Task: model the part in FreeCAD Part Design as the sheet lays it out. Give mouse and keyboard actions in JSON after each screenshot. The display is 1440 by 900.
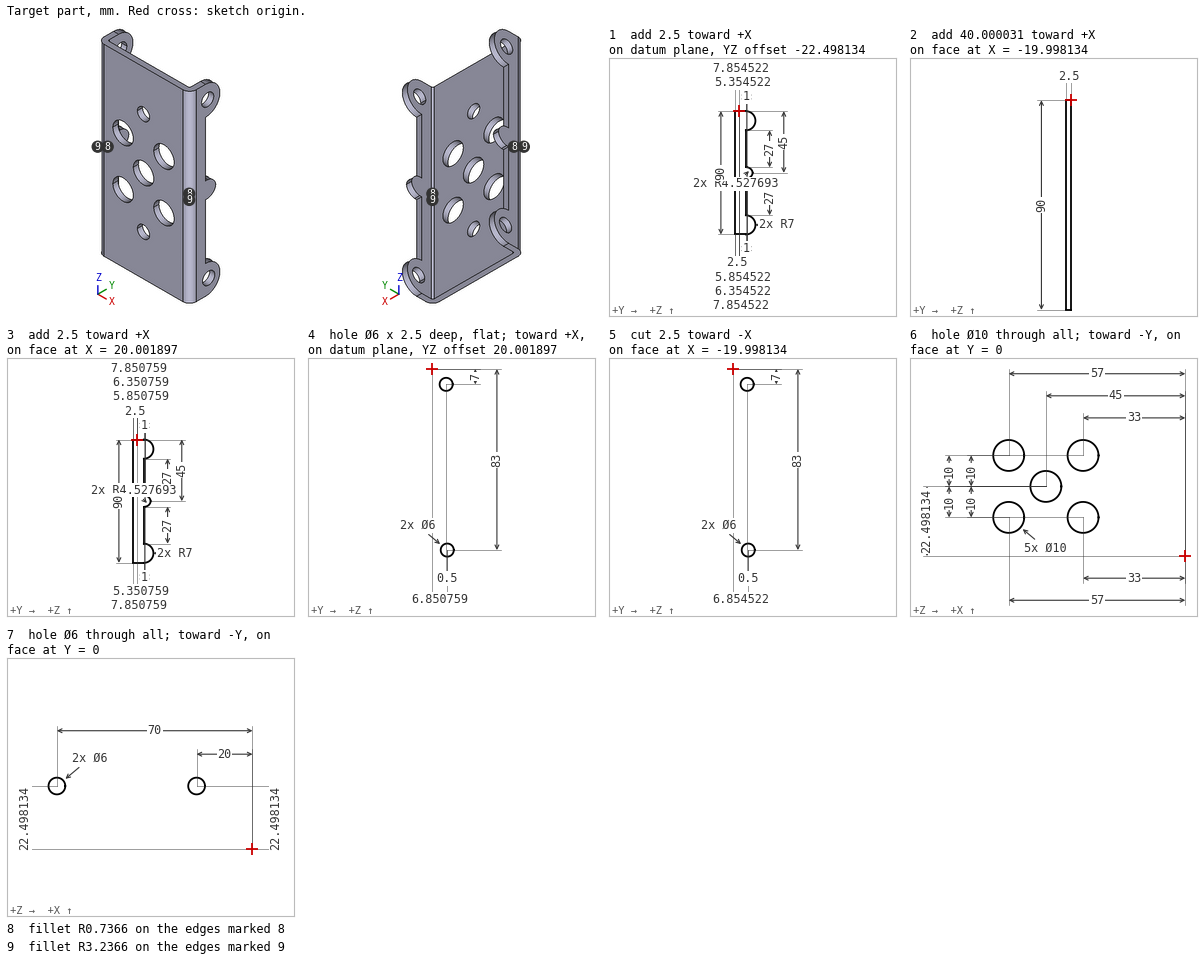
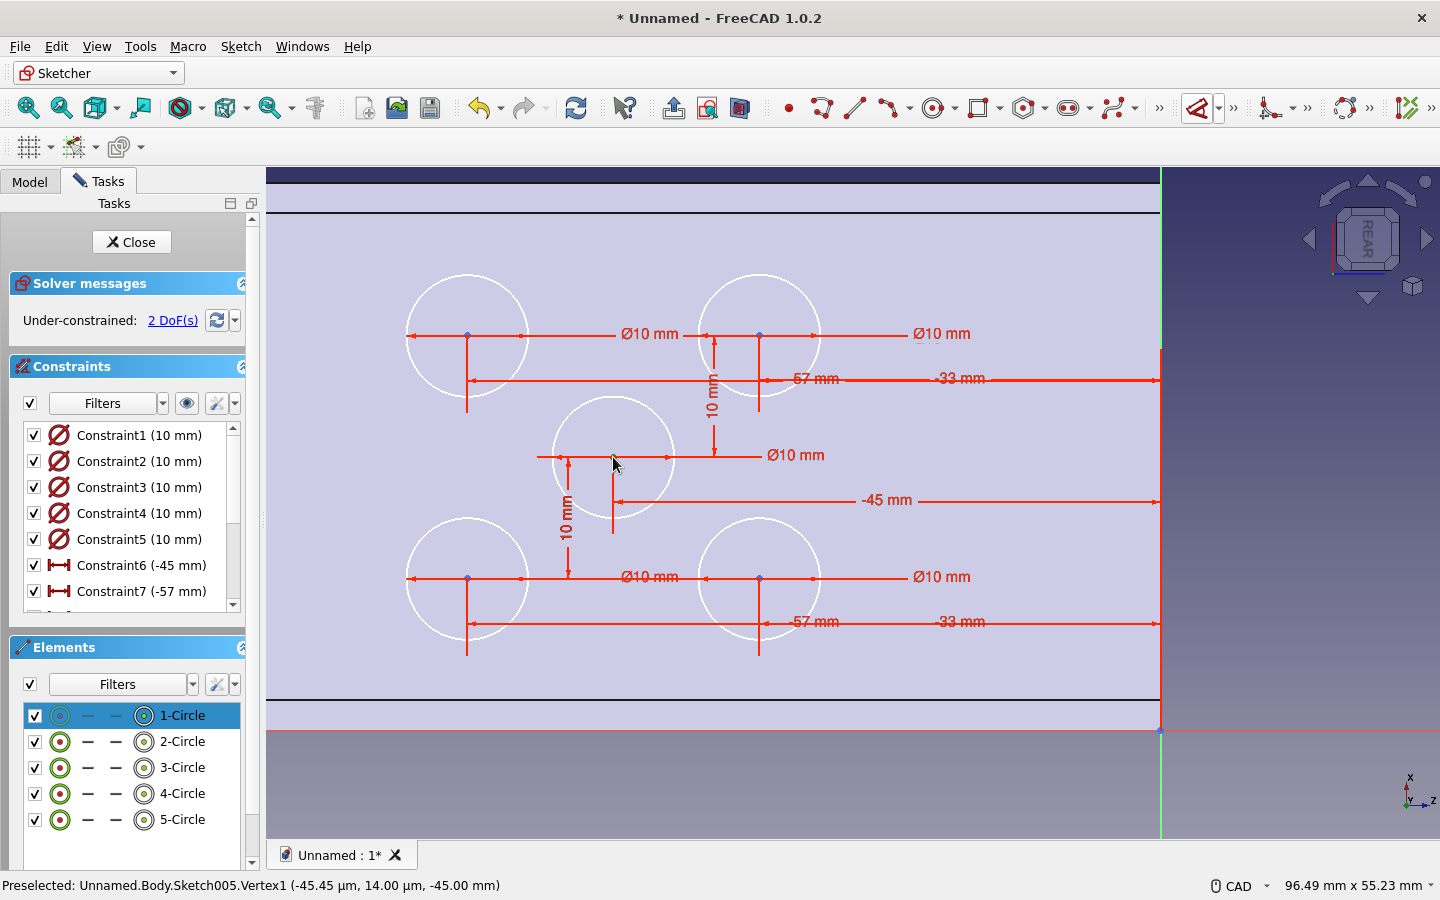
{"action": "left_click", "coordinate": [467, 336]}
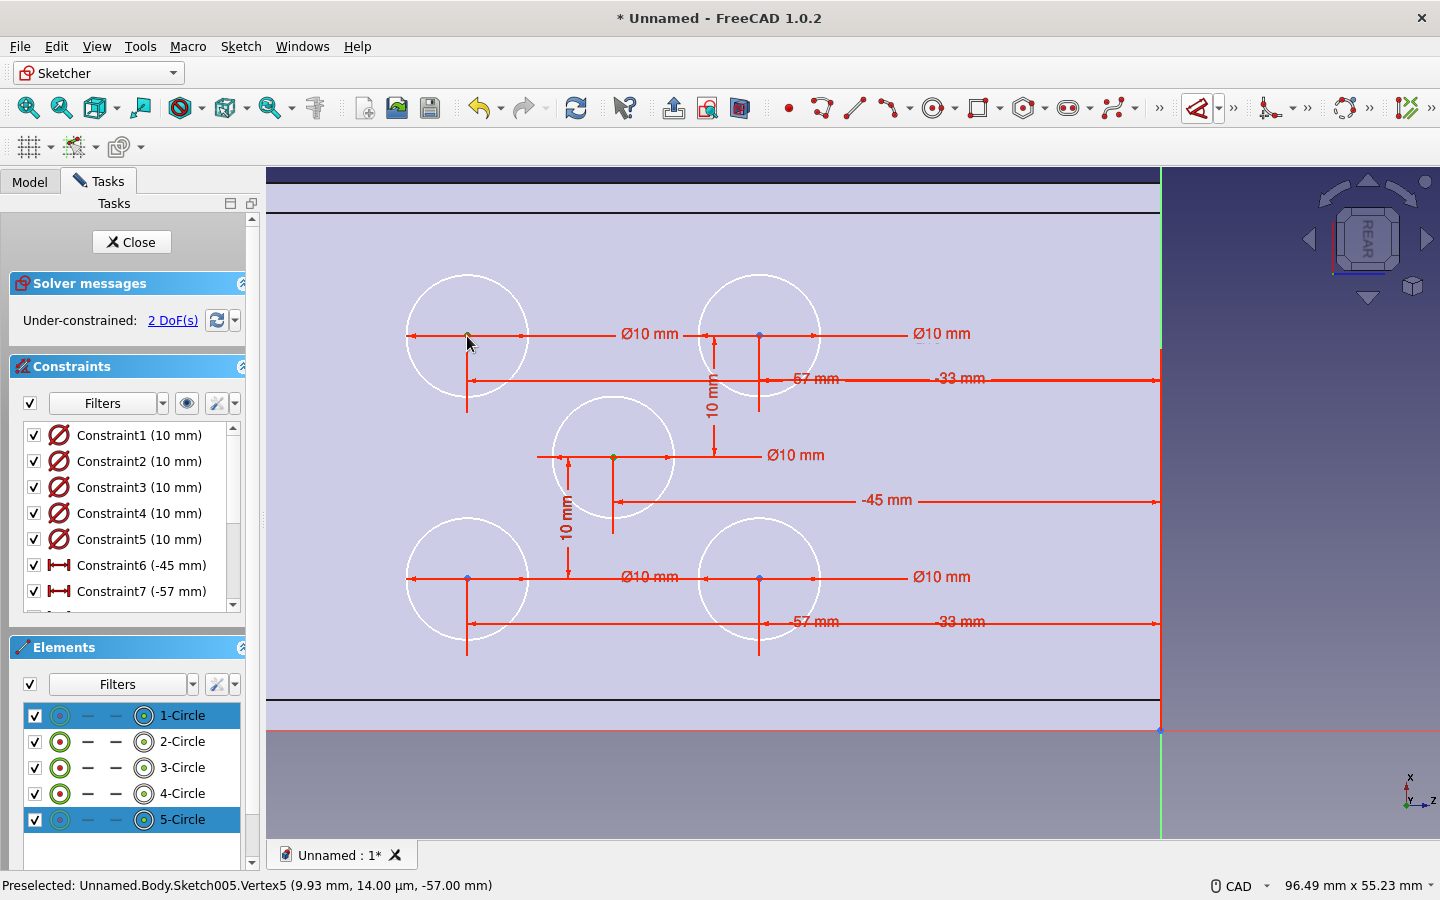
{"action": "key", "text": "i"}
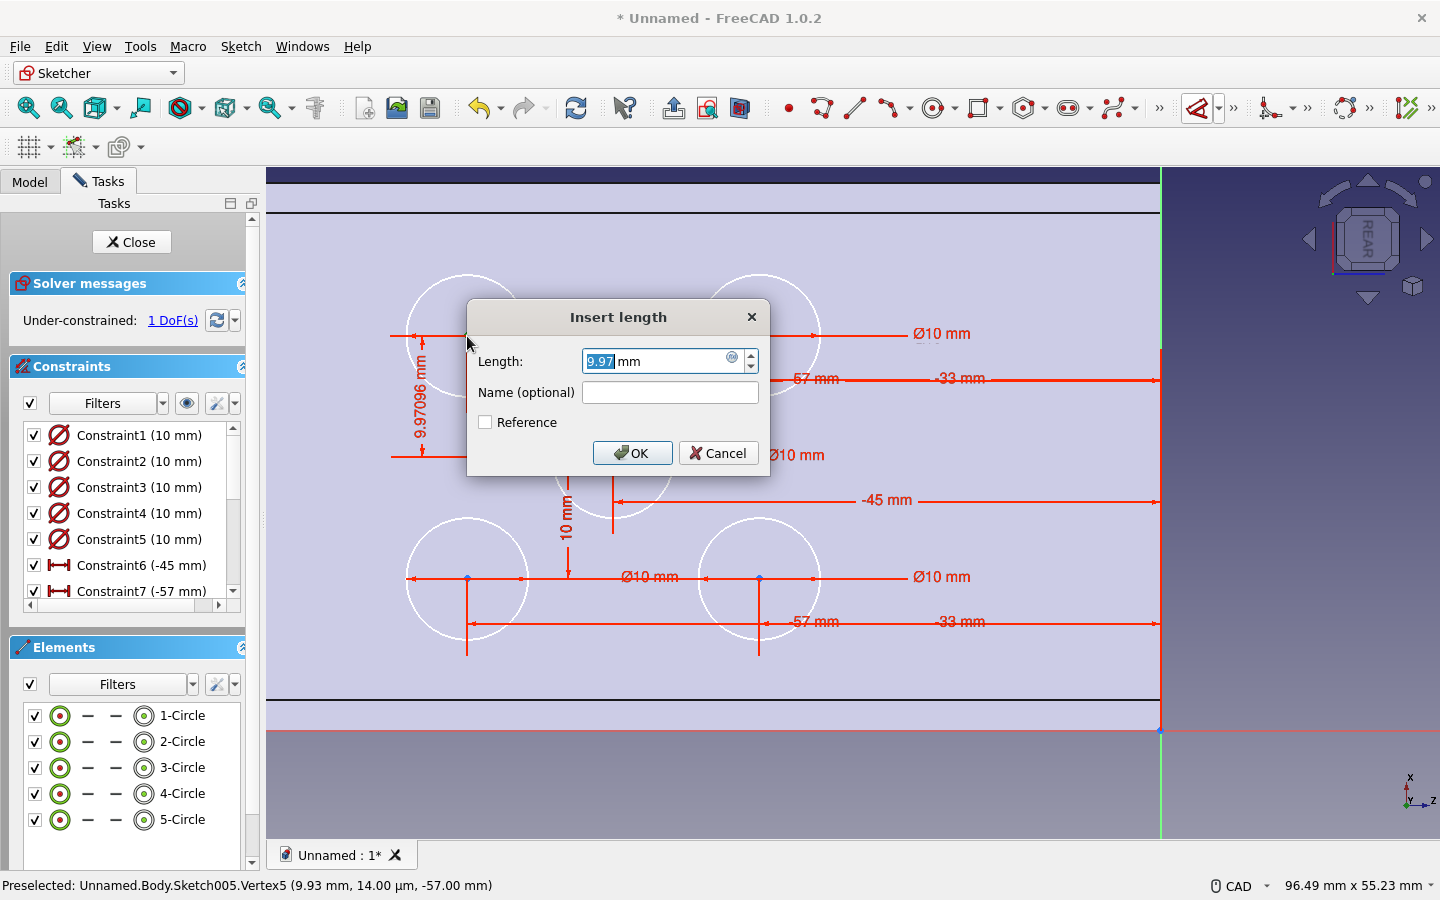
{"action": "type", "text": "10"}
{"action": "key", "text": "Return"}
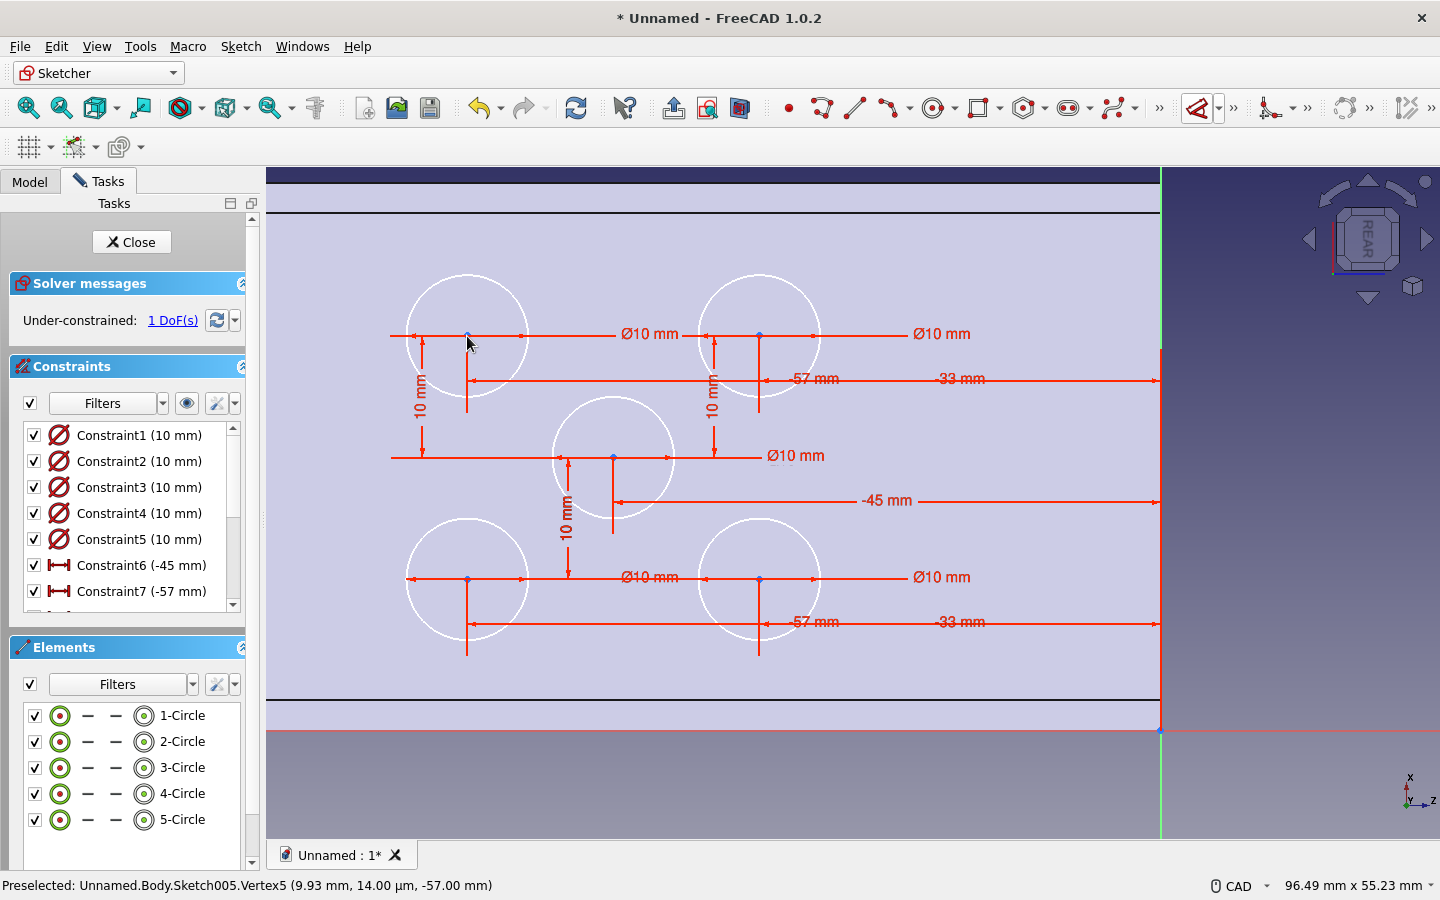
{"action": "left_click", "coordinate": [613, 458]}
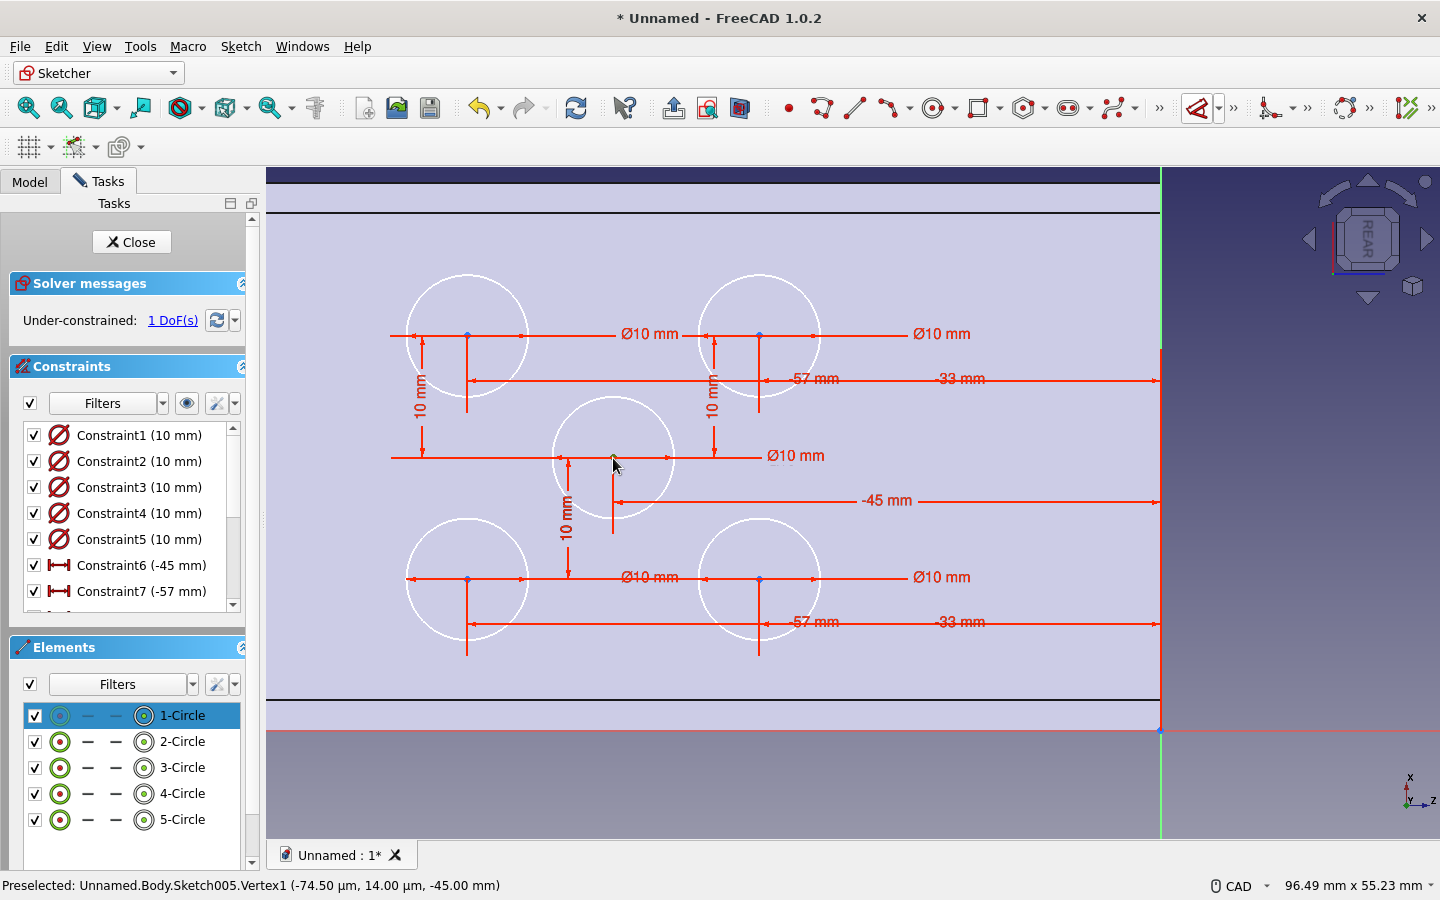
{"action": "left_click", "coordinate": [1218, 108]}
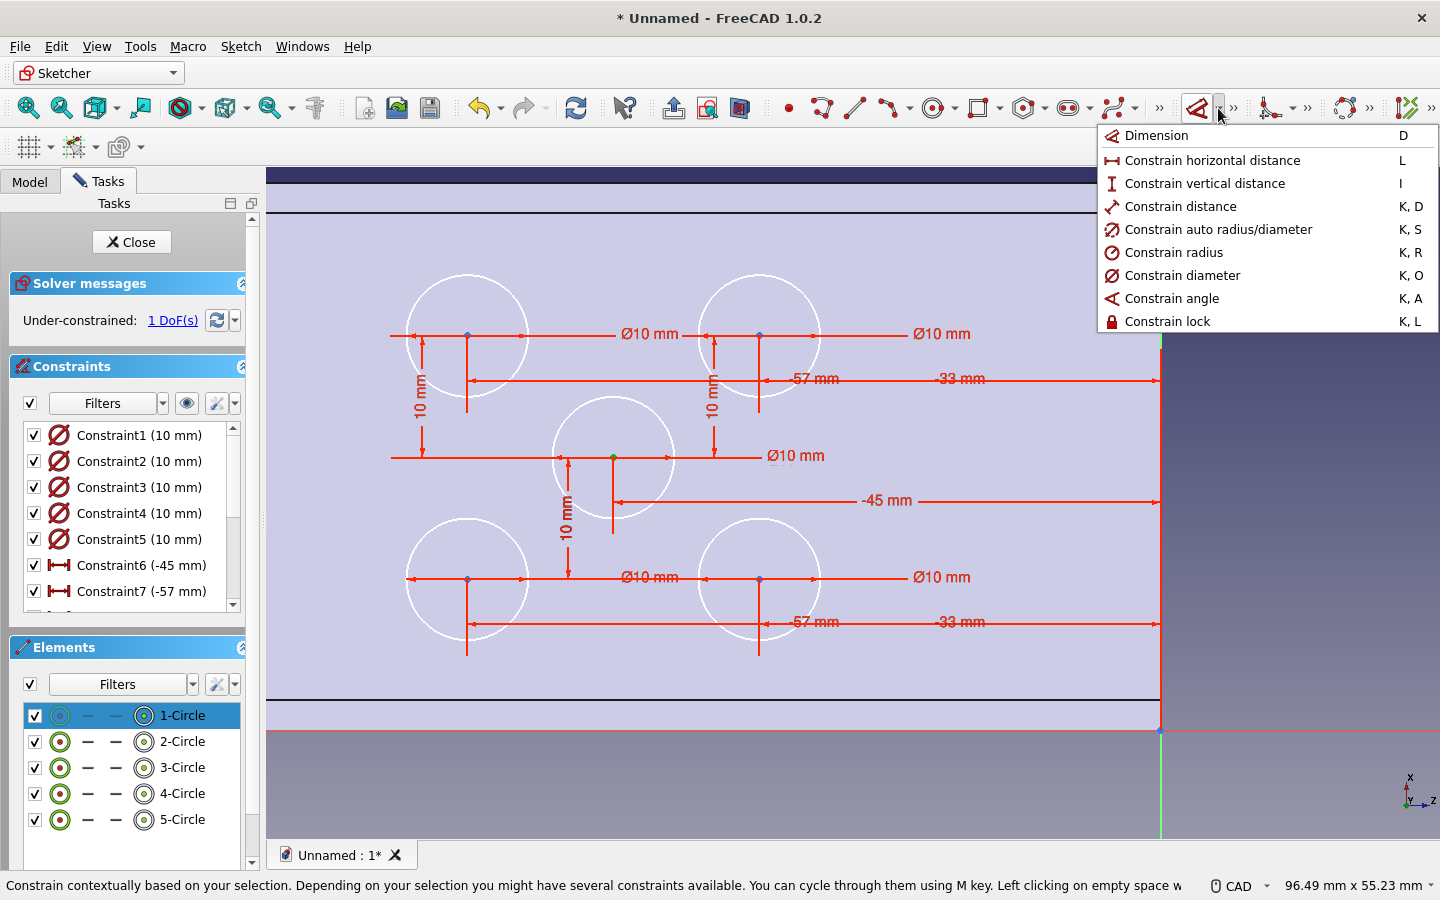
{"action": "left_click", "coordinate": [1268, 184]}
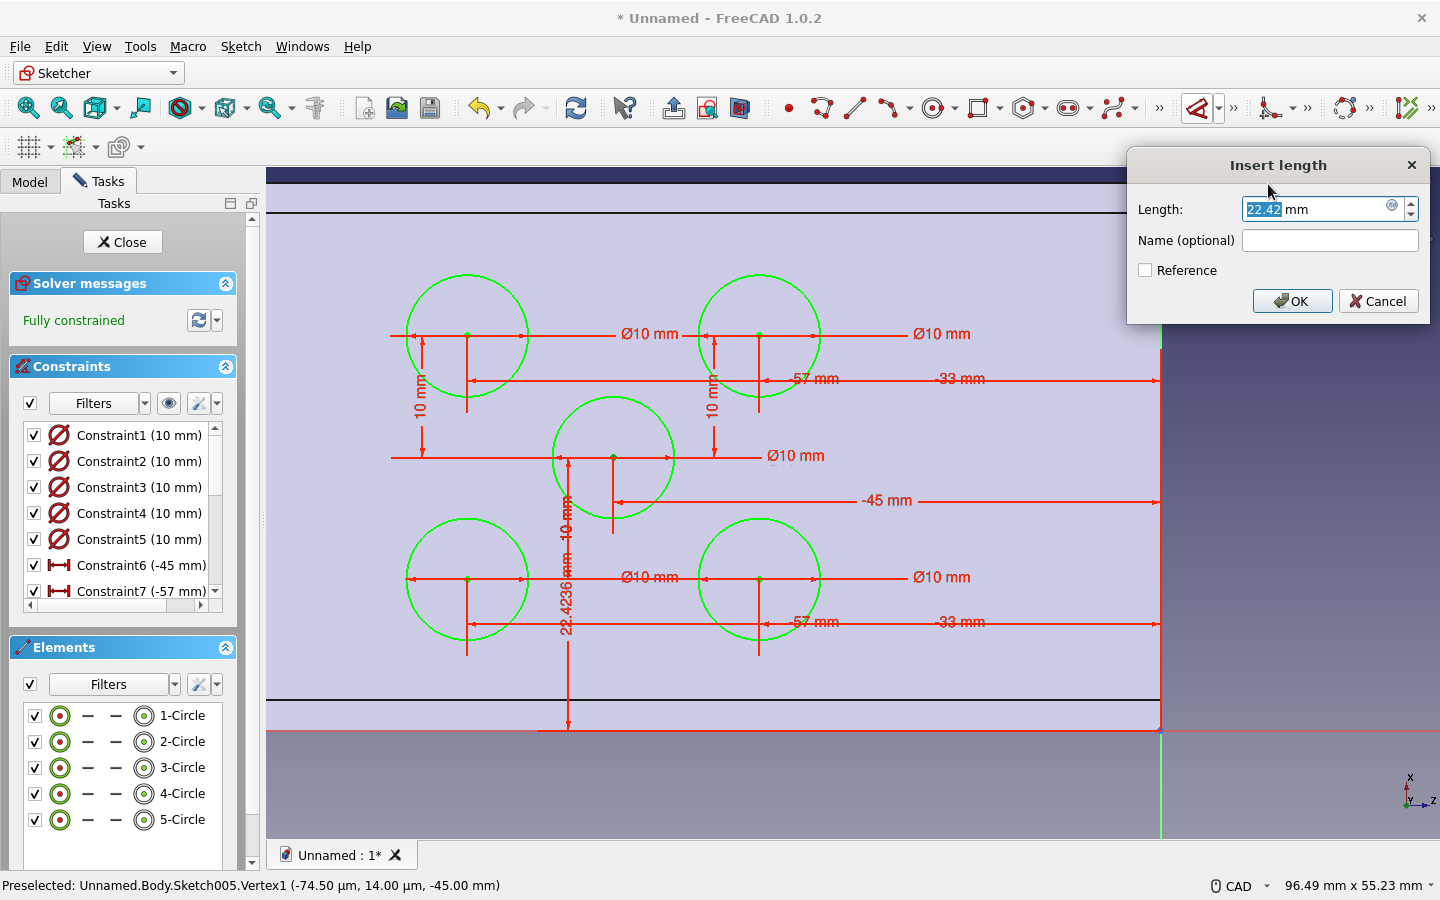
{"action": "type", "text": "22.498134"}
{"action": "key", "text": "Return"}